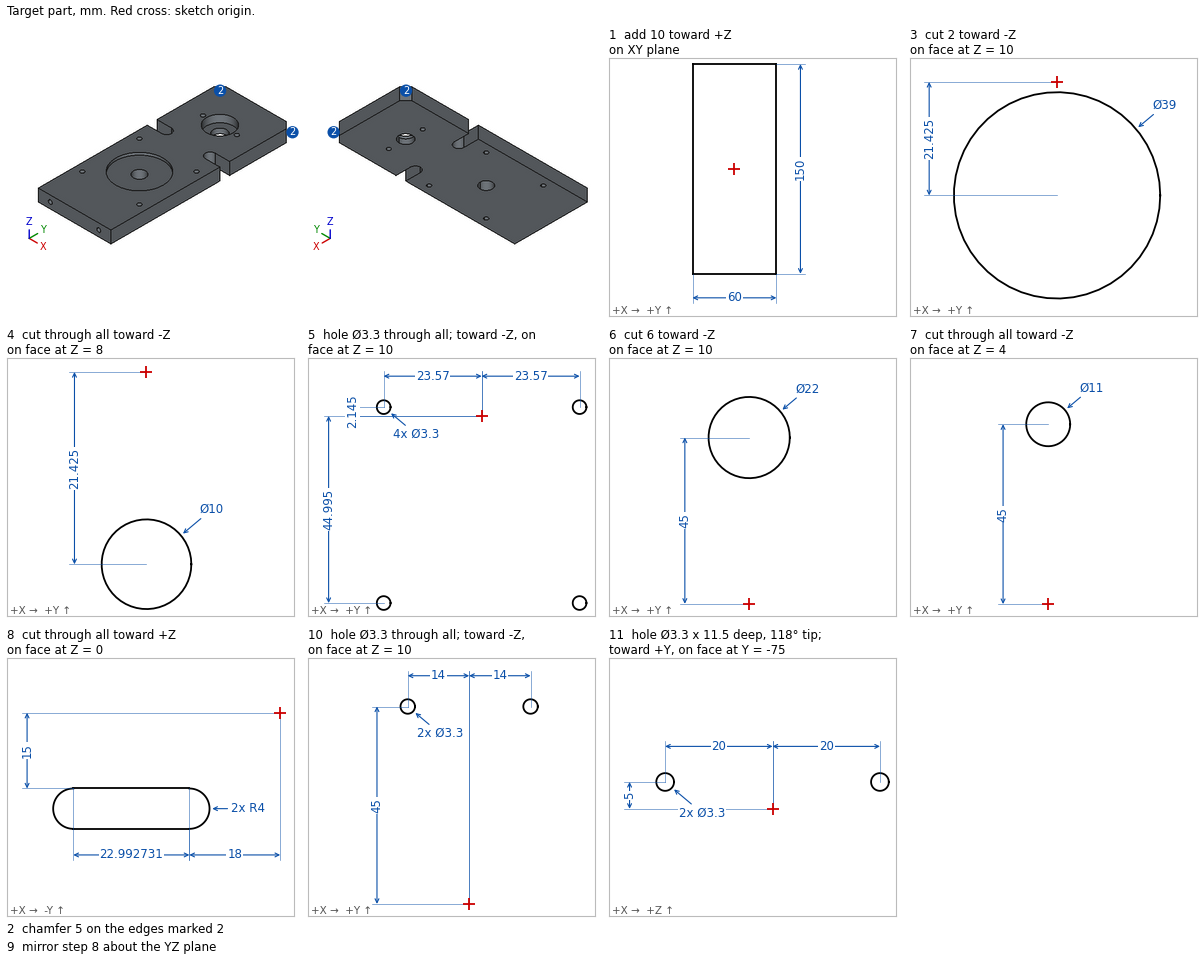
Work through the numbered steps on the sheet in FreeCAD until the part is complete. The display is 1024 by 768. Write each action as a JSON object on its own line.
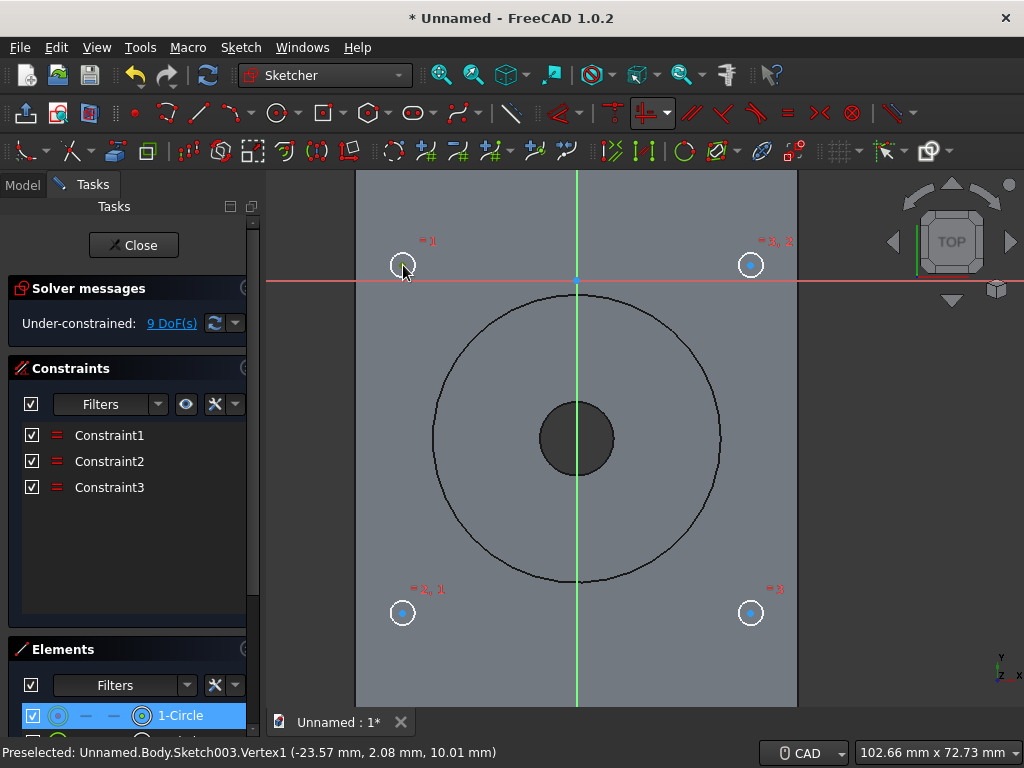
{"action": "left_click", "coordinate": [403, 613]}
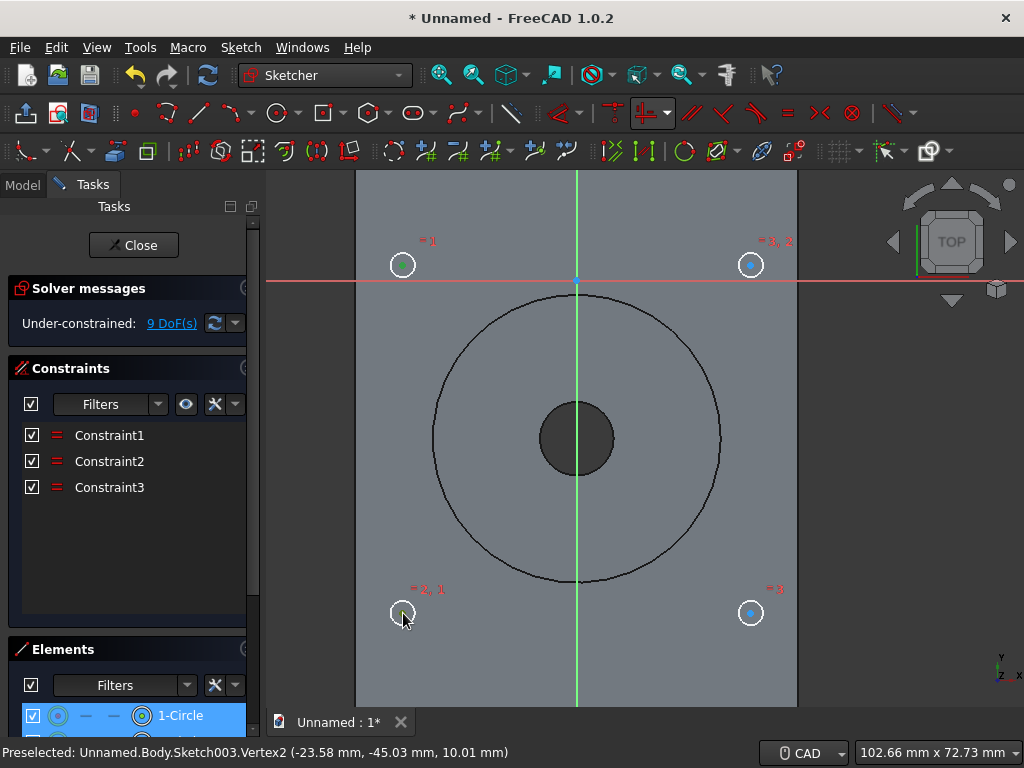
{"action": "key", "text": "v"}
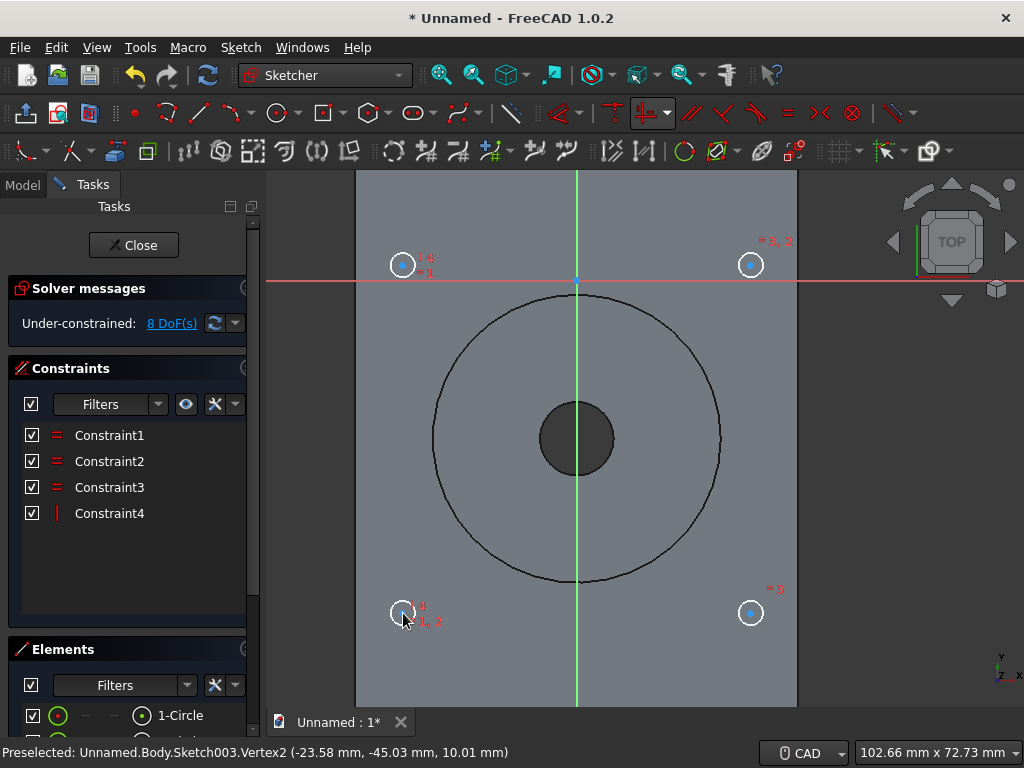
{"action": "left_click", "coordinate": [403, 265]}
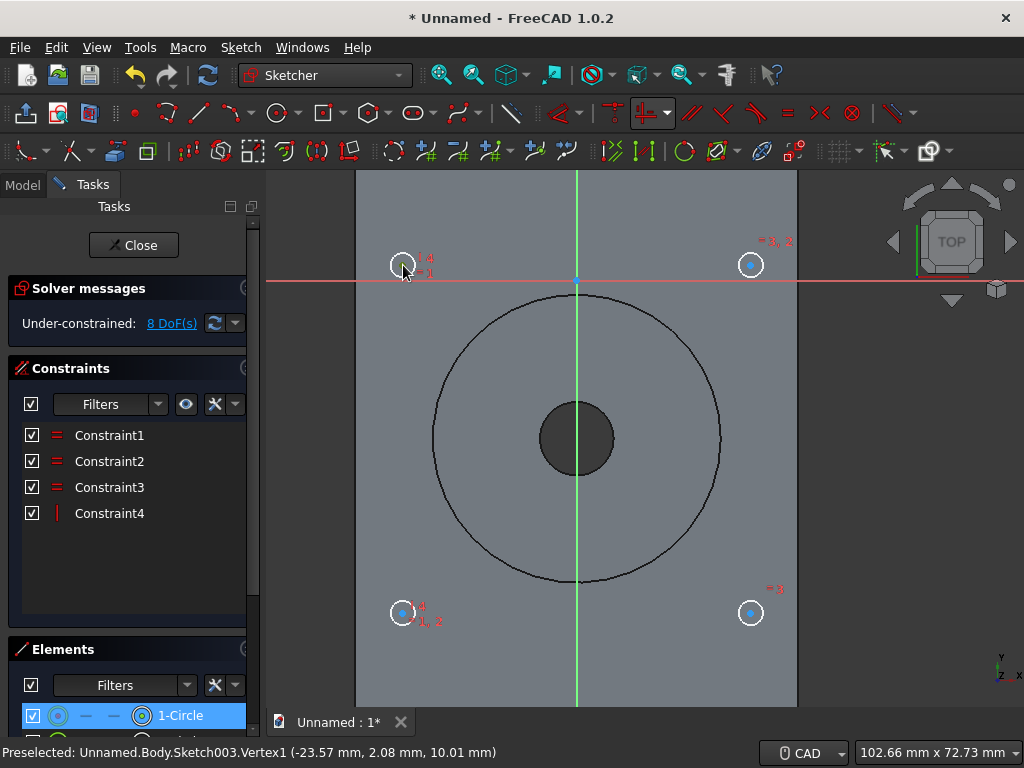
{"action": "left_click", "coordinate": [751, 265]}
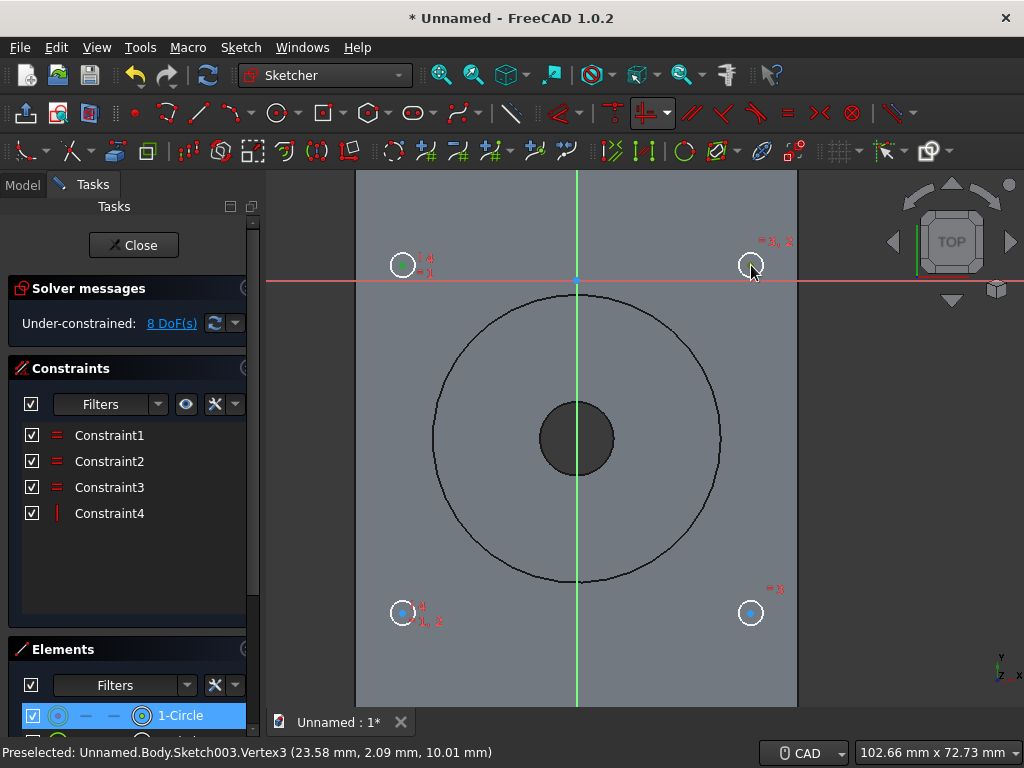
{"action": "key", "text": "h"}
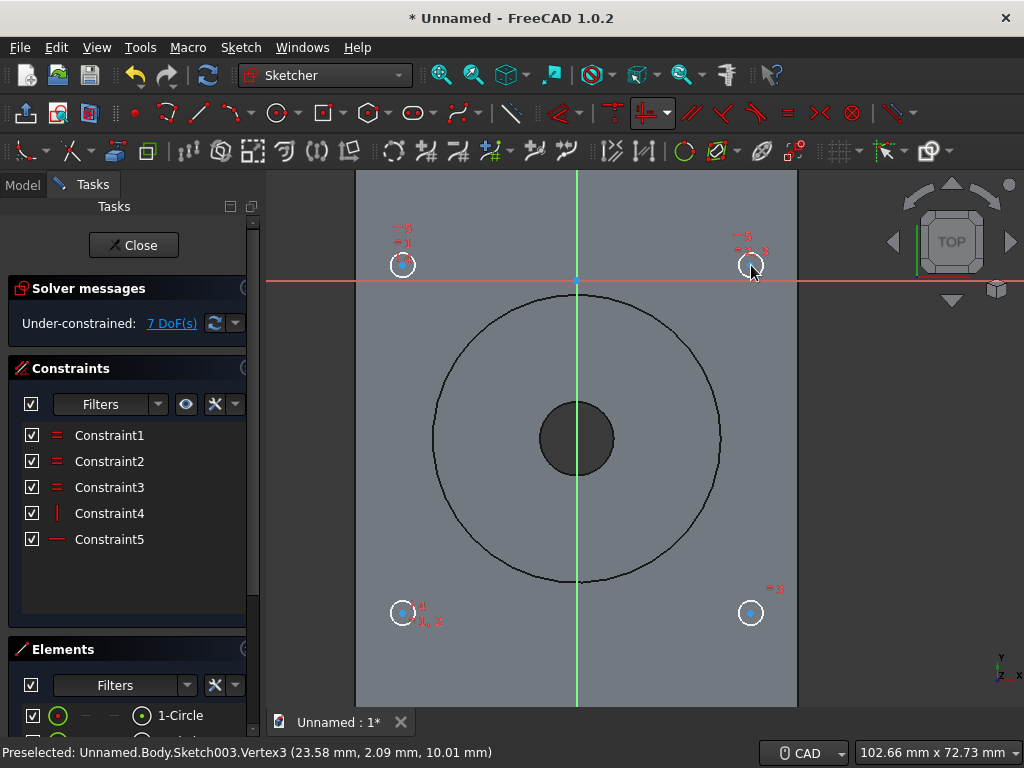
{"action": "left_click", "coordinate": [751, 265]}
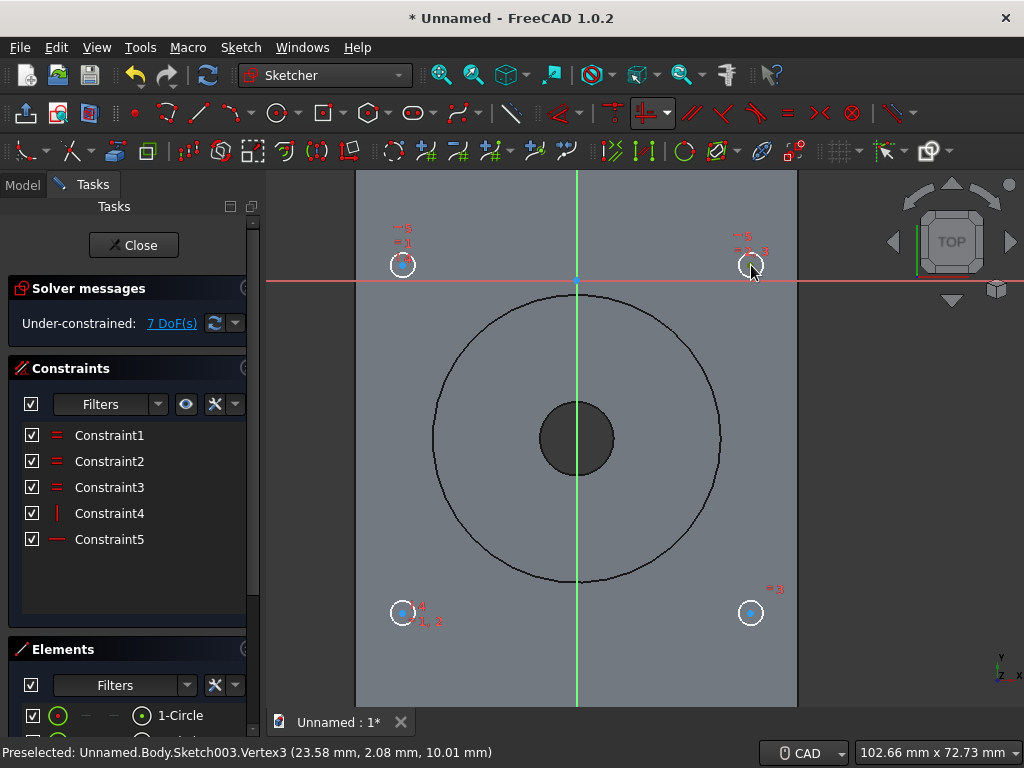
{"action": "left_click", "coordinate": [751, 613]}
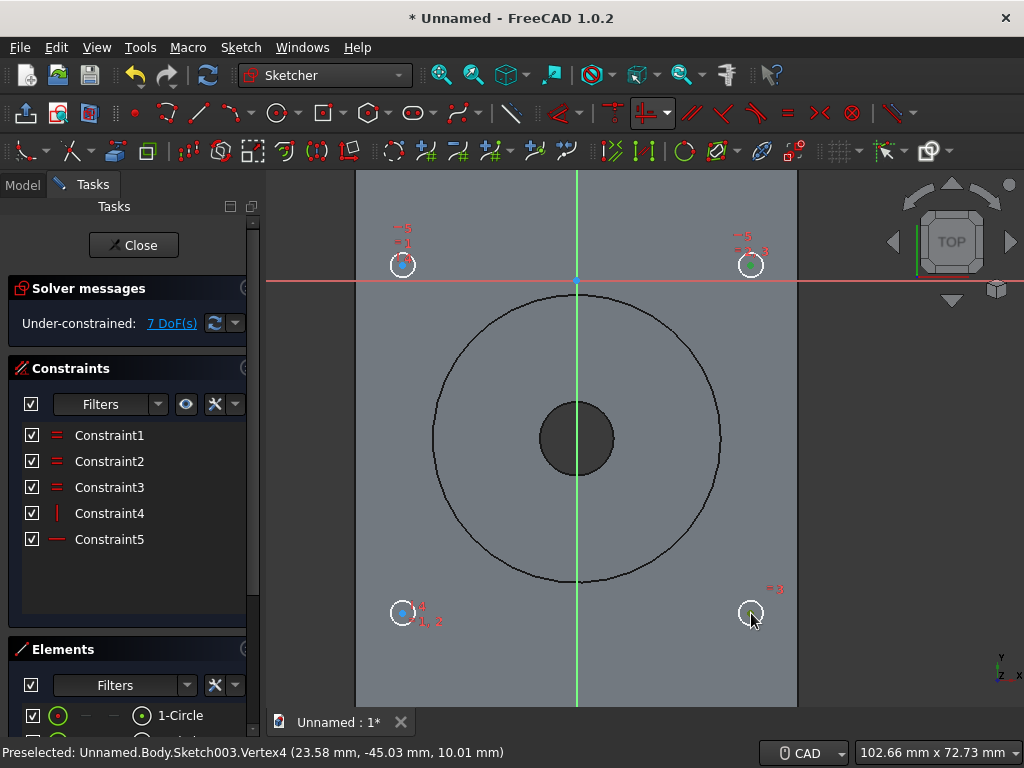
{"action": "left_click", "coordinate": [670, 114]}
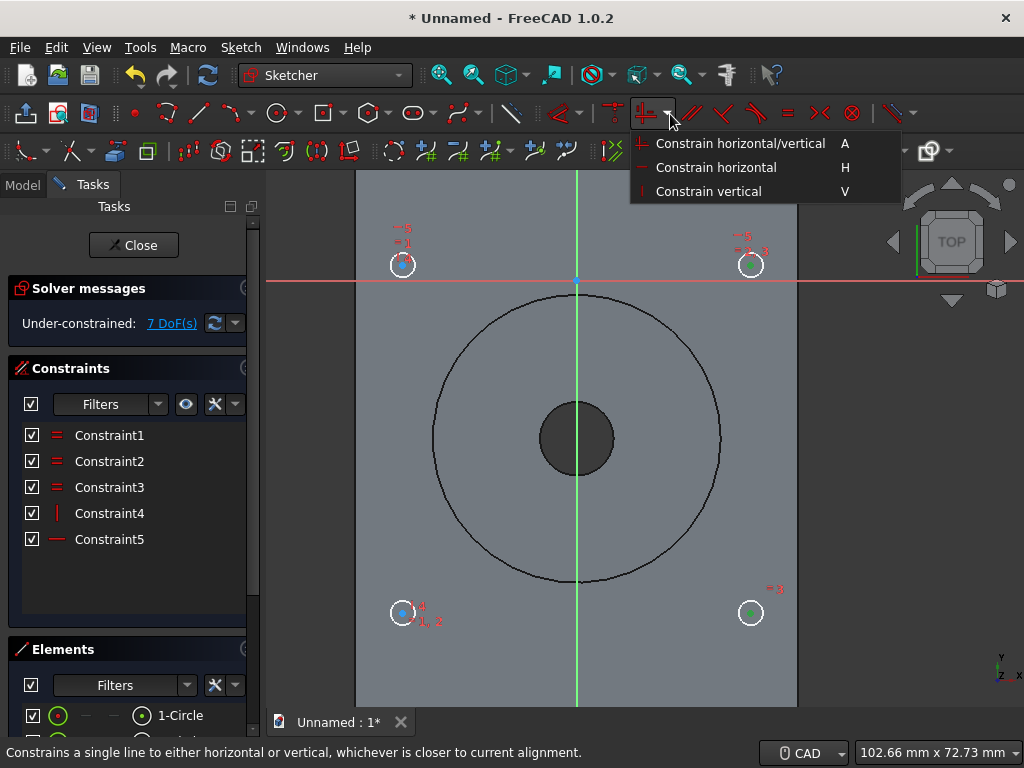
{"action": "left_click", "coordinate": [766, 191]}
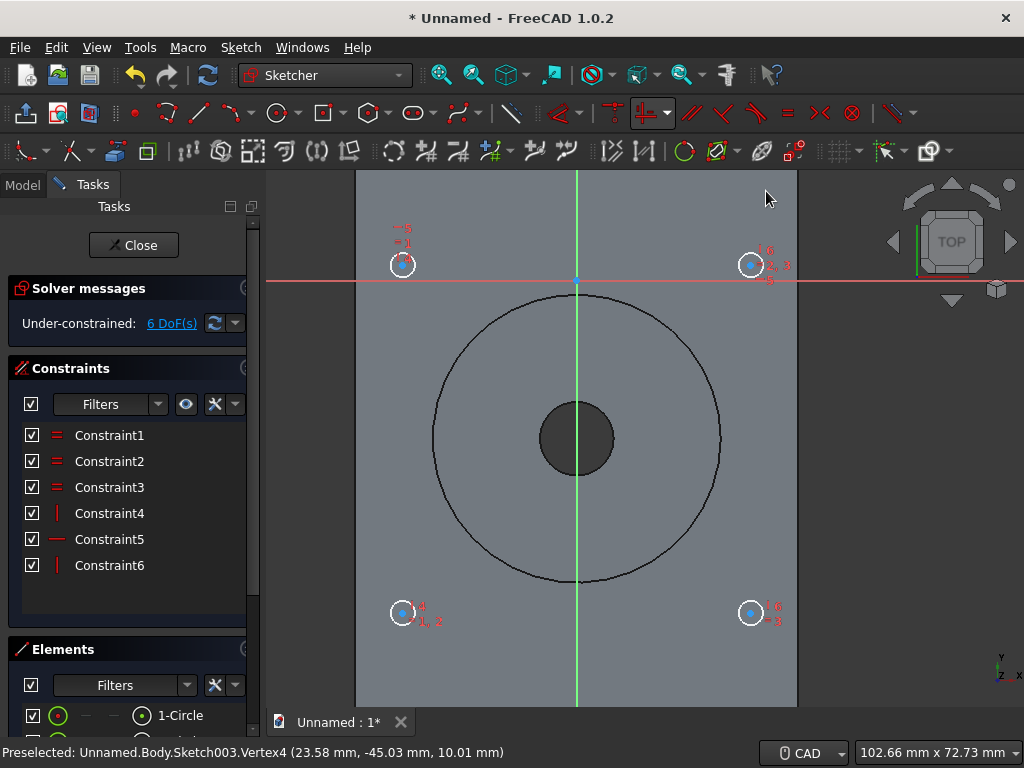
{"action": "left_click", "coordinate": [403, 613]}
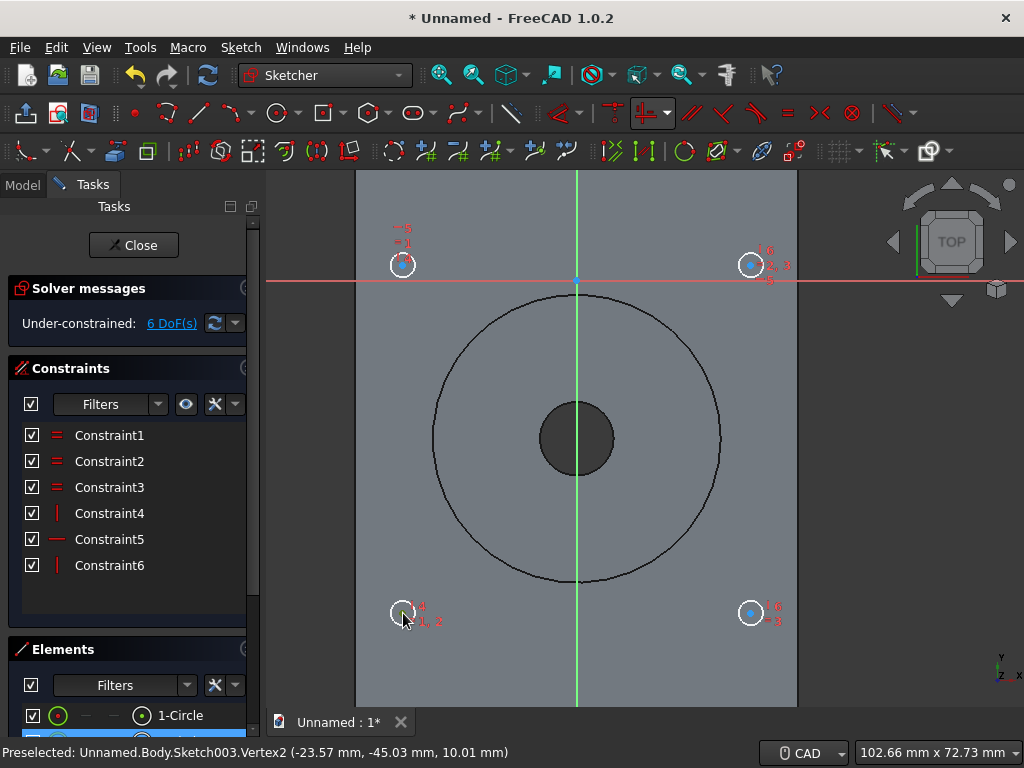
{"action": "left_click", "coordinate": [751, 613]}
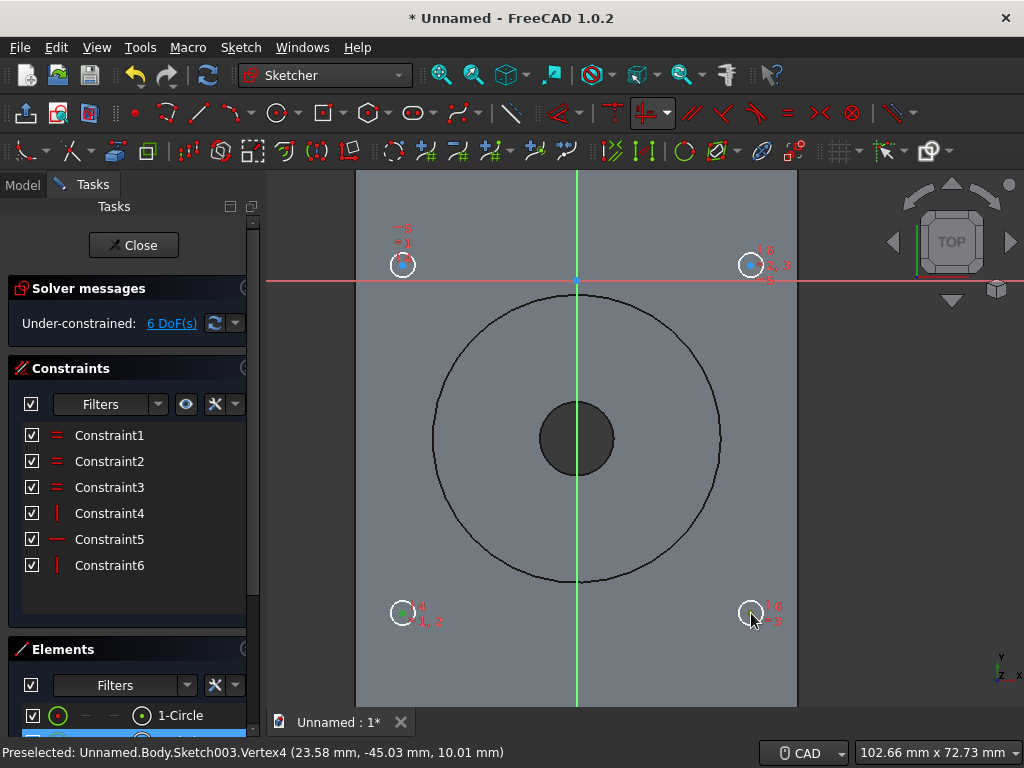
{"action": "left_click", "coordinate": [670, 114]}